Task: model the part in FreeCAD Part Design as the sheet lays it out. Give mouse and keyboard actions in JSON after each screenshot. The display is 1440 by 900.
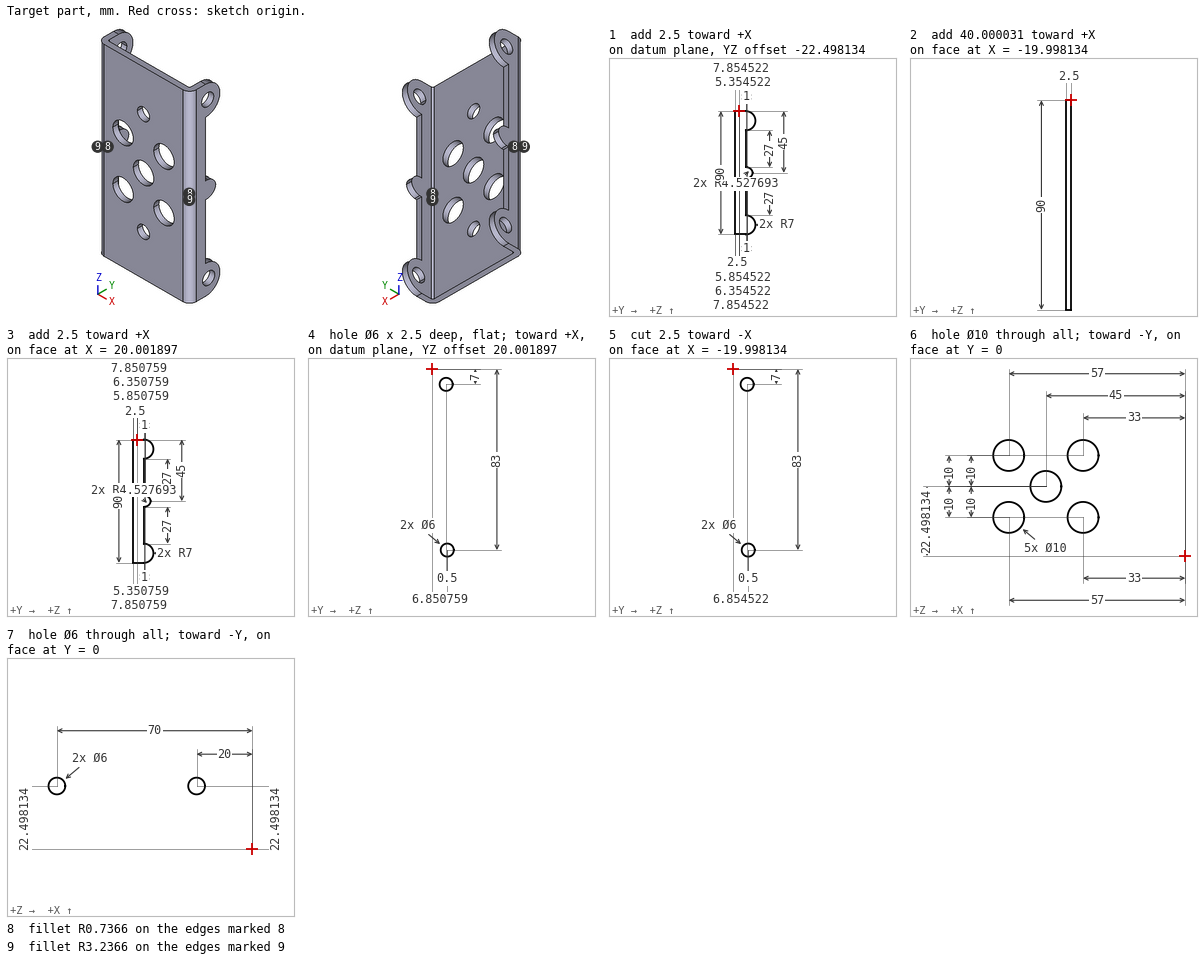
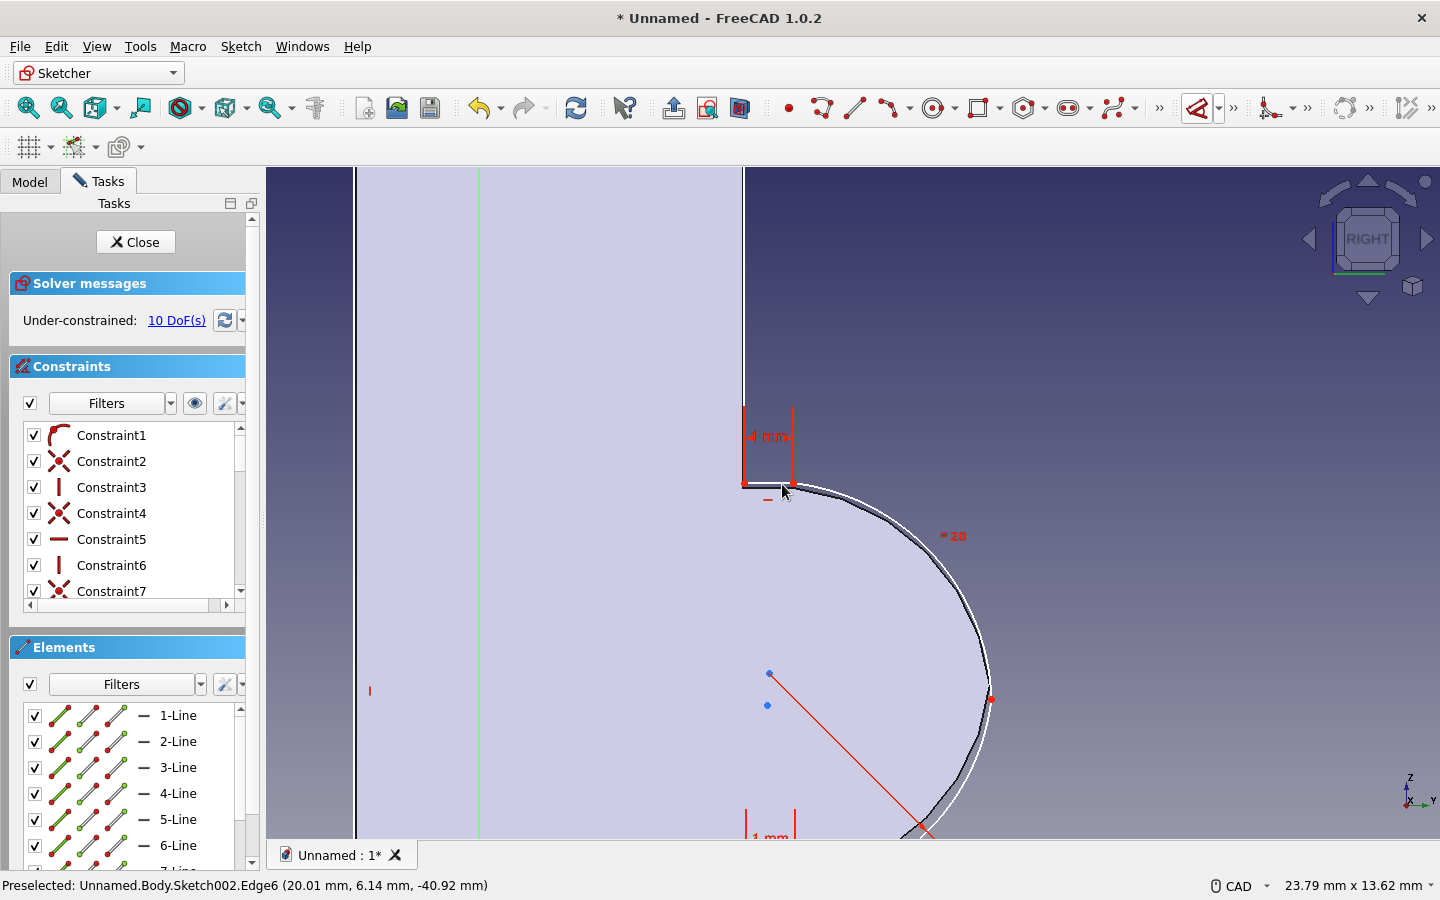
{"action": "scroll", "coordinate": [791, 485], "scroll_direction": "down", "scroll_amount": 12}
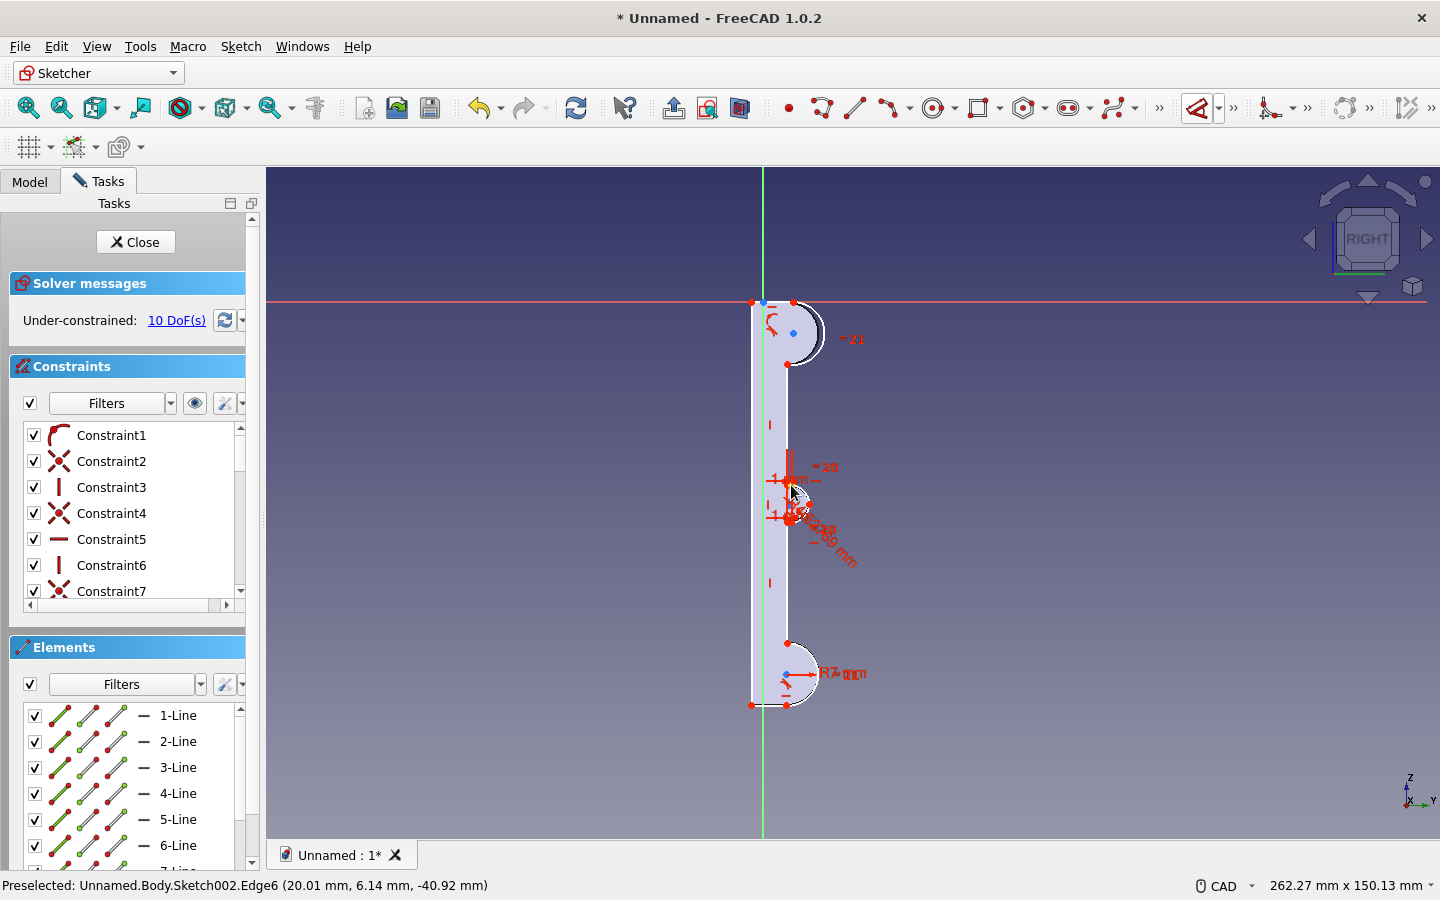
{"action": "left_click", "coordinate": [752, 464]}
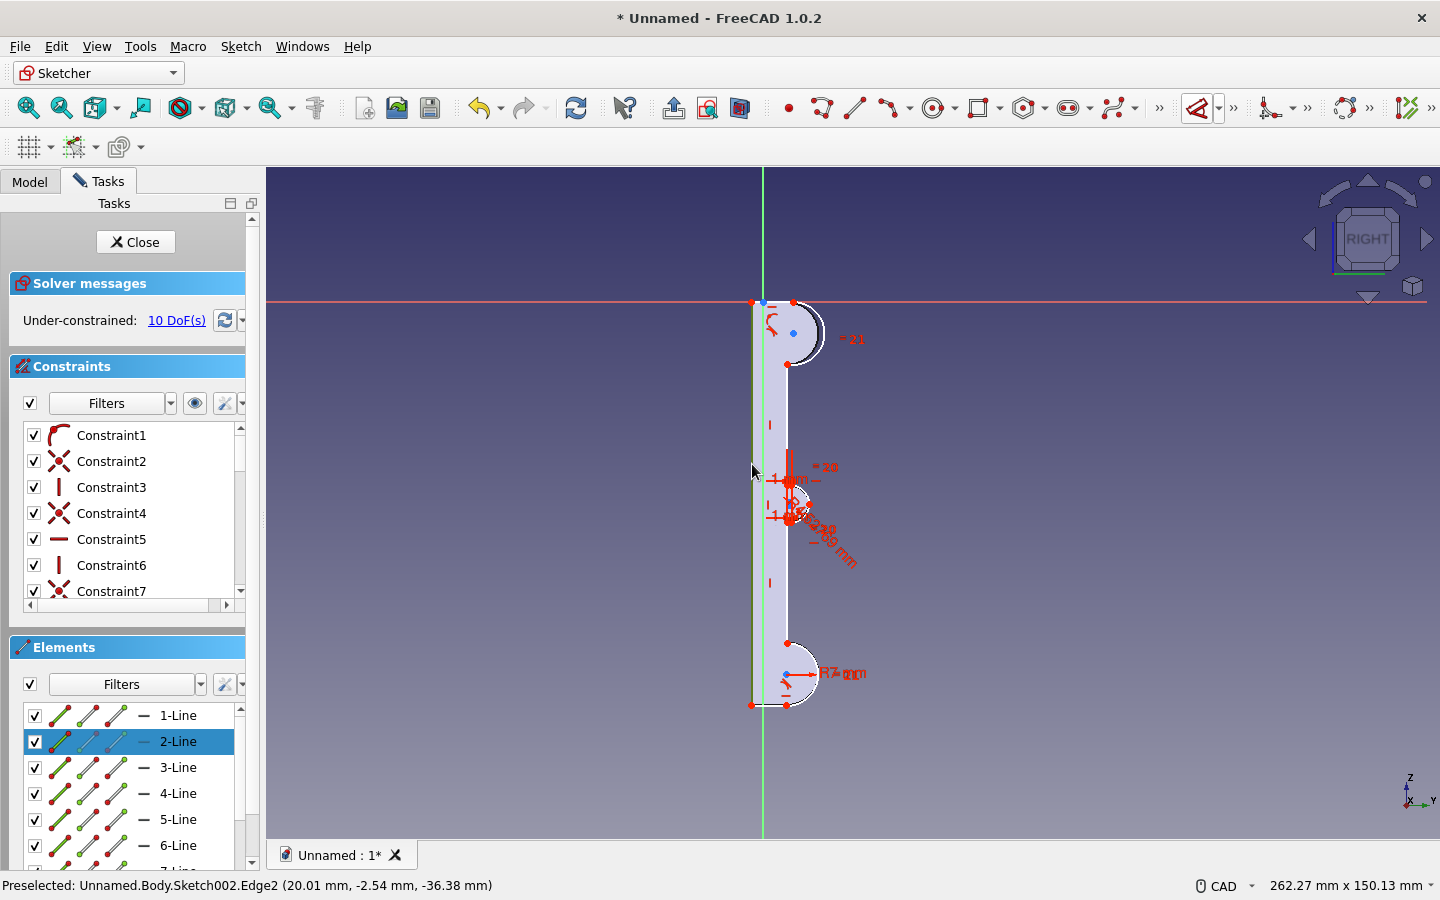
{"action": "left_click", "coordinate": [1218, 108]}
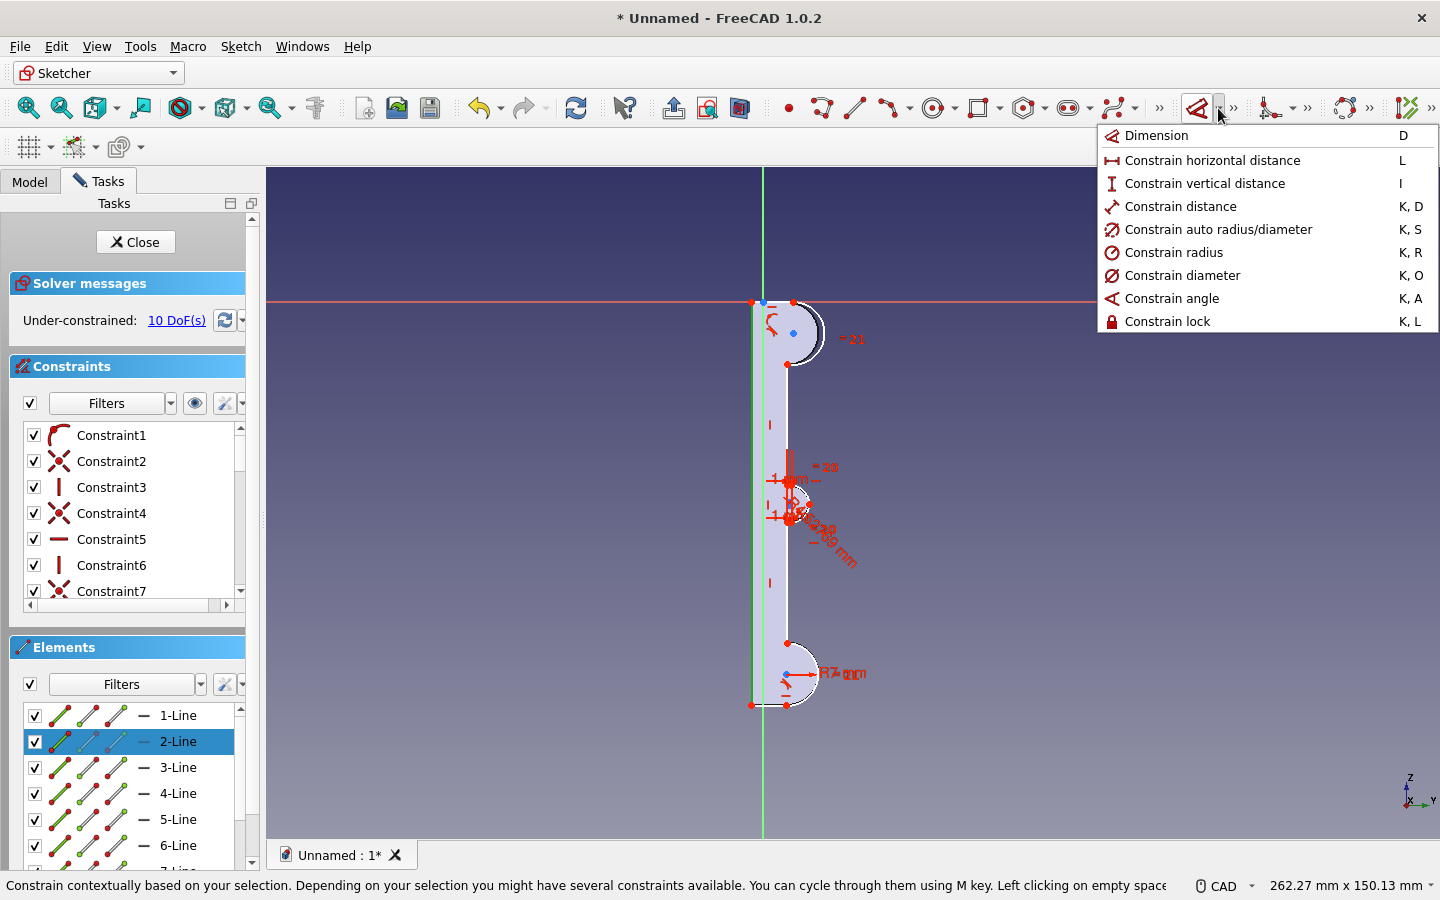
{"action": "left_click", "coordinate": [1268, 184]}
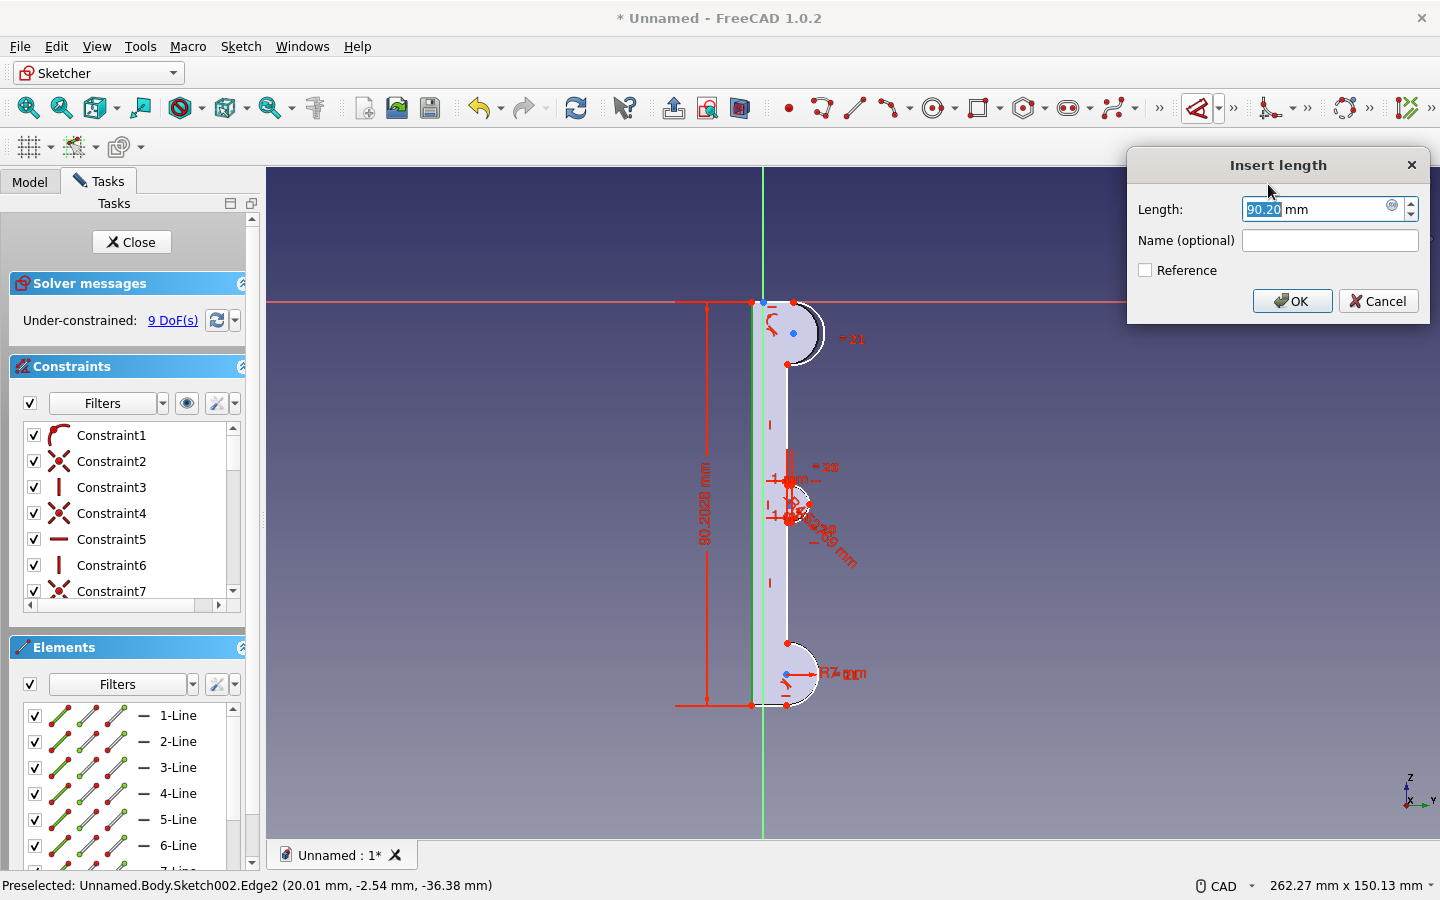
{"action": "type", "text": "90"}
{"action": "key", "text": "Return"}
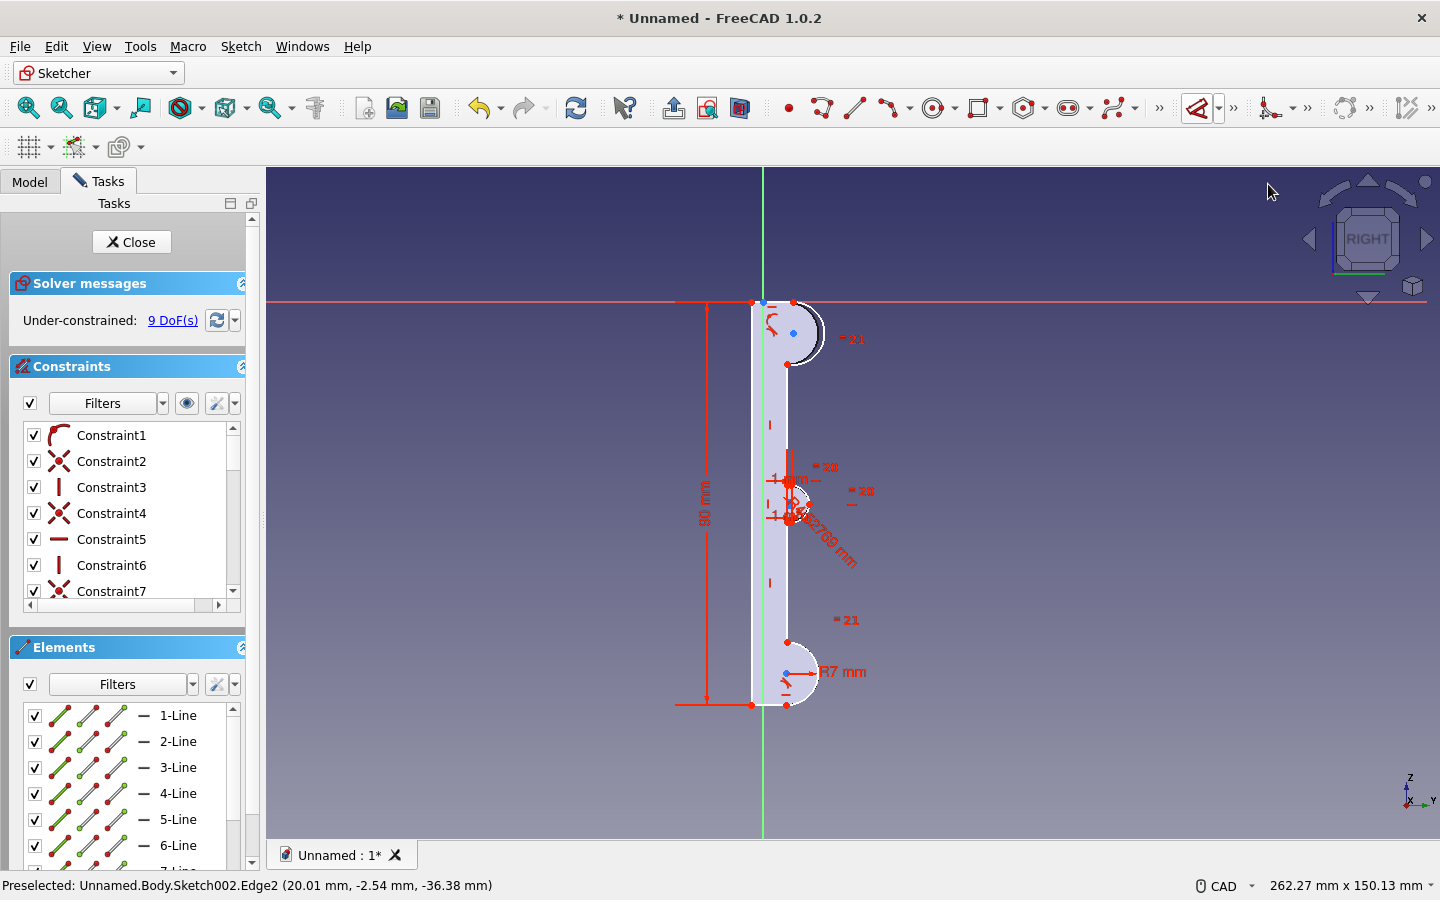
{"action": "left_click", "coordinate": [787, 606]}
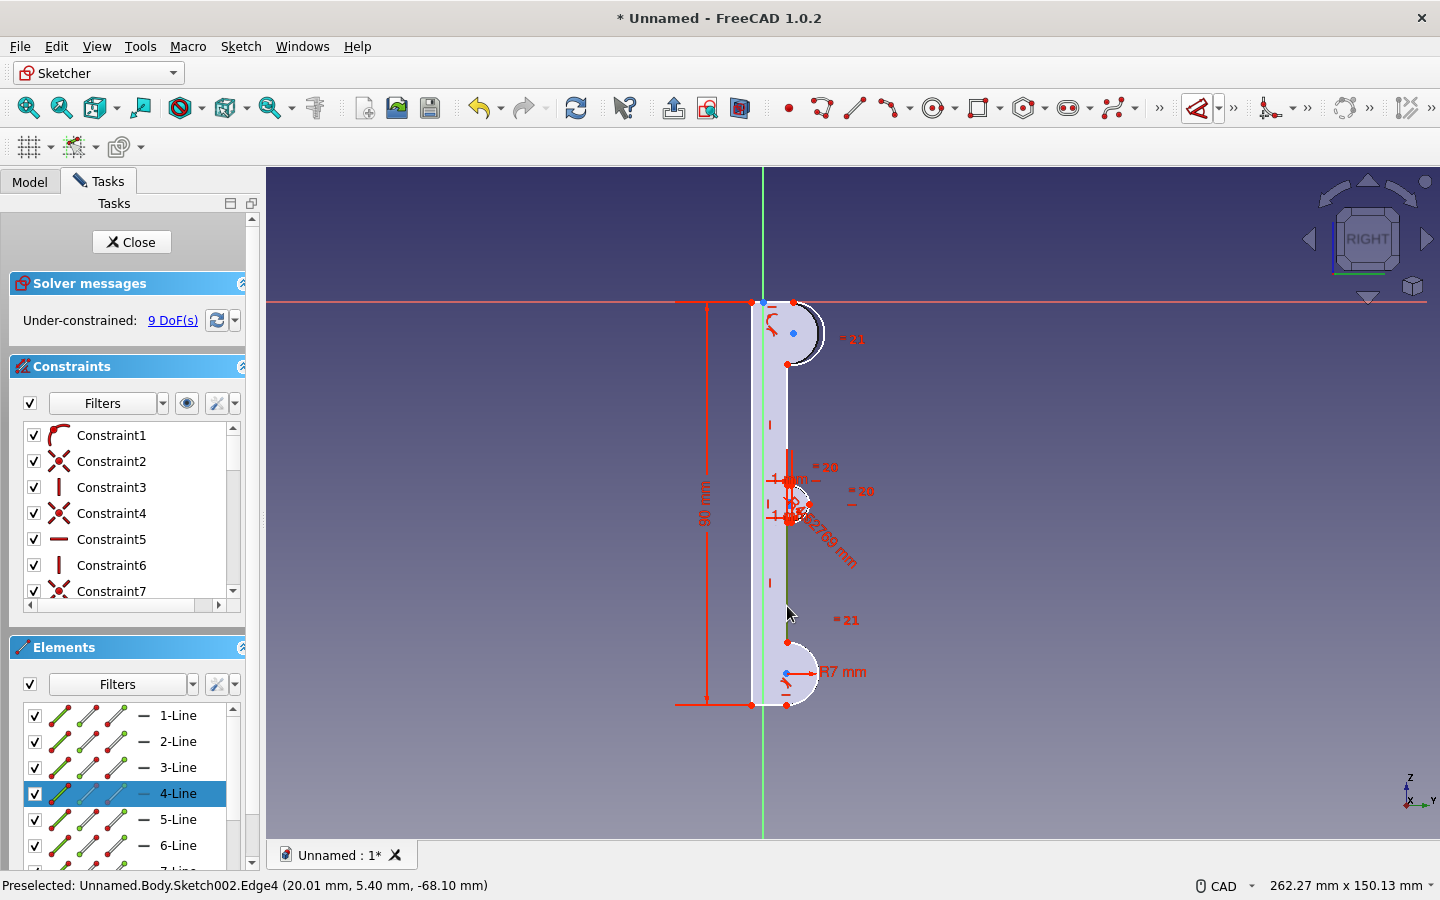
{"action": "left_click", "coordinate": [1218, 108]}